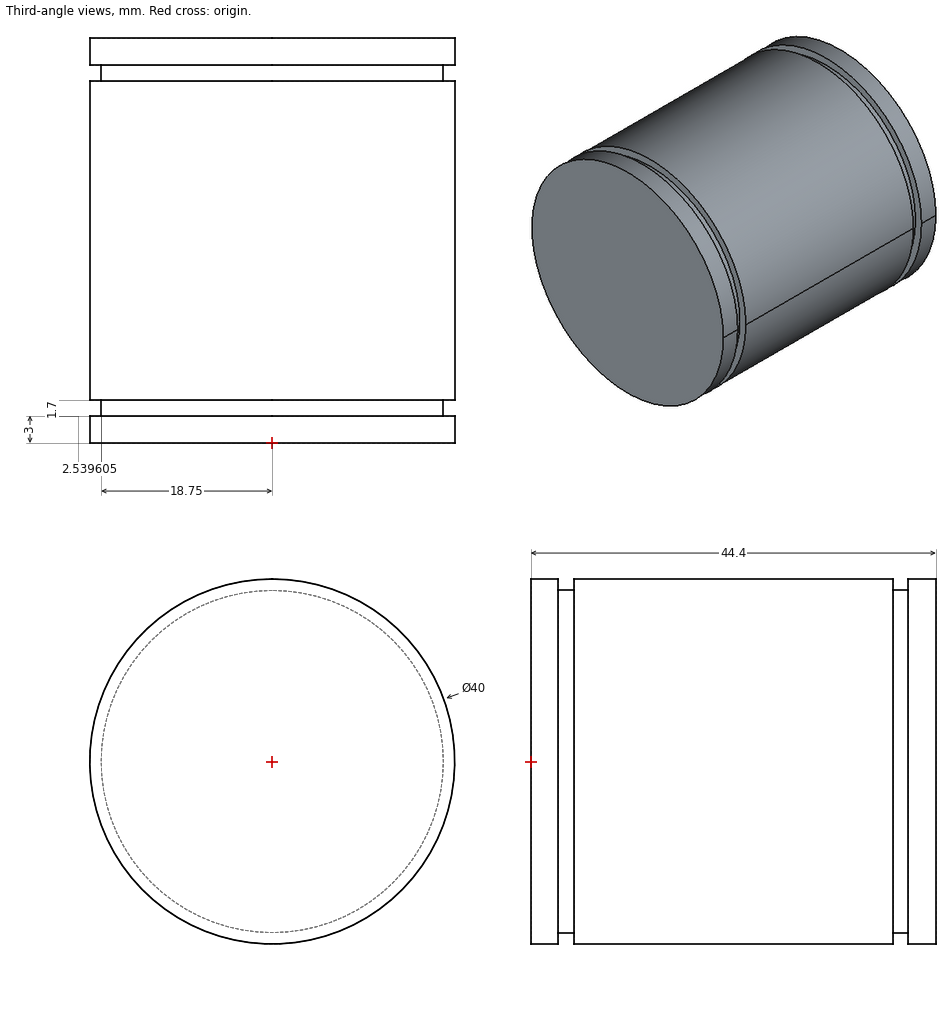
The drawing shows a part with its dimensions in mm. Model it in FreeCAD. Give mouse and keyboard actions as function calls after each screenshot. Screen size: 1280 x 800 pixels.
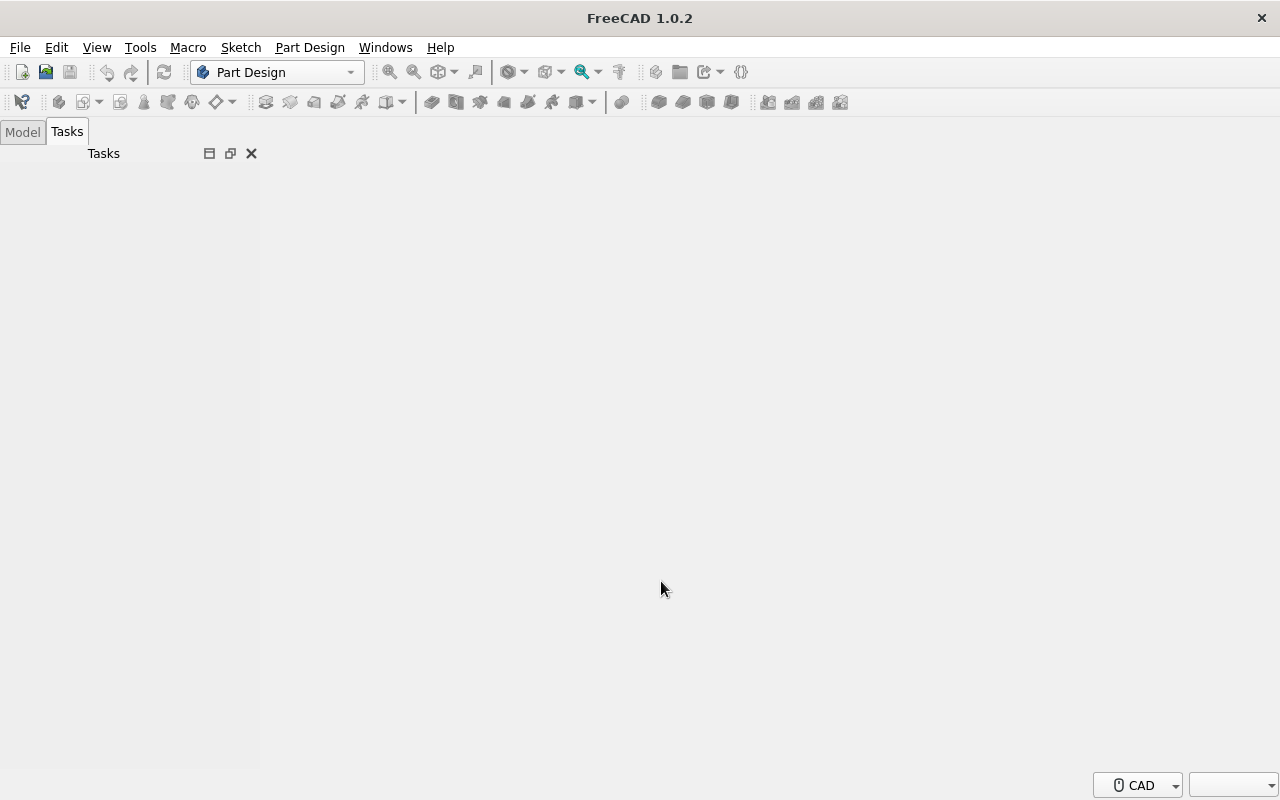
key(ctrl+n)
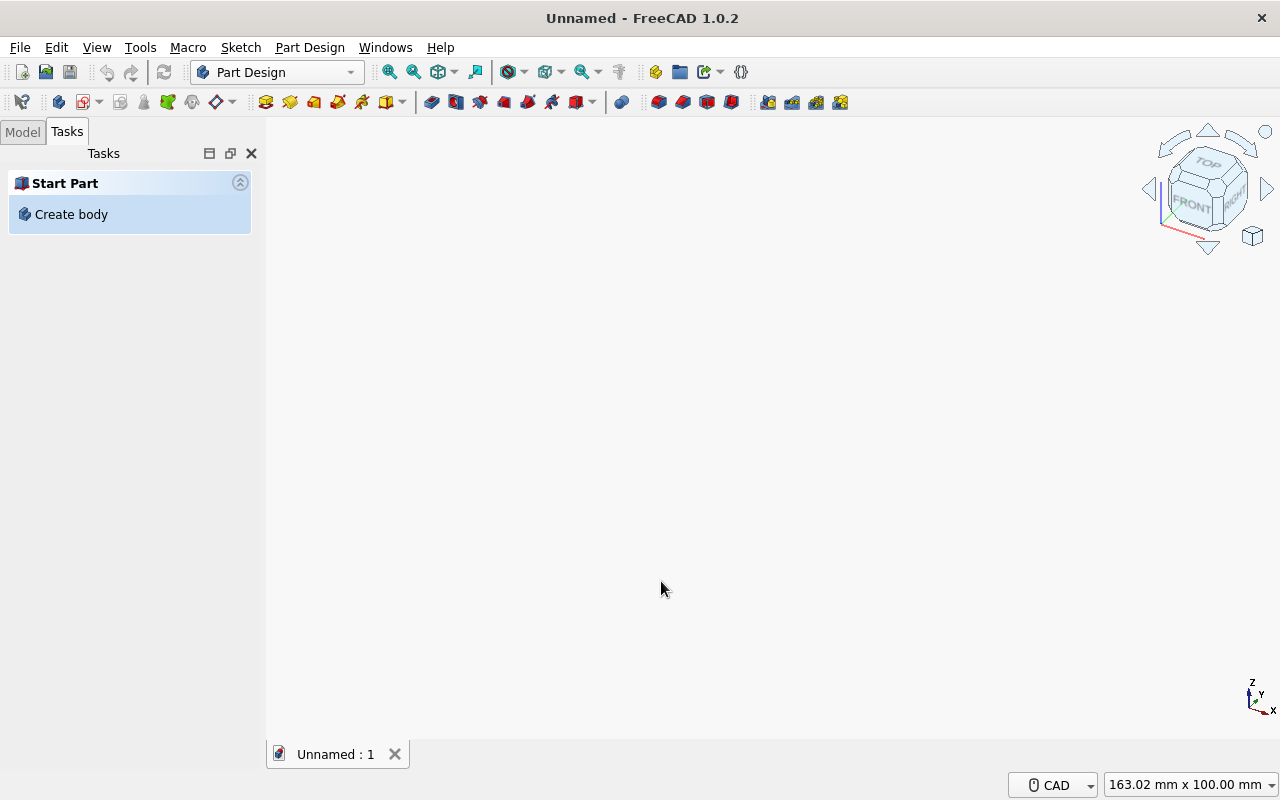
click(84, 102)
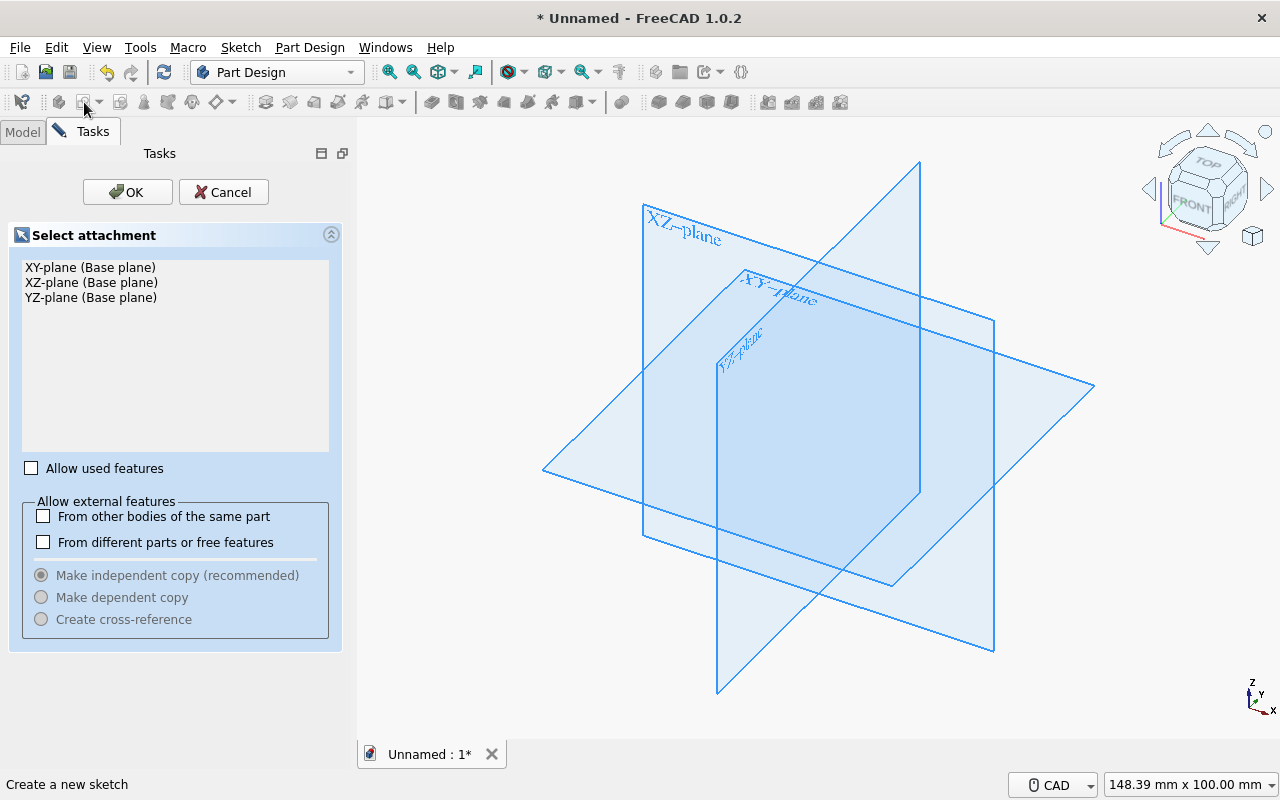
click(82, 282)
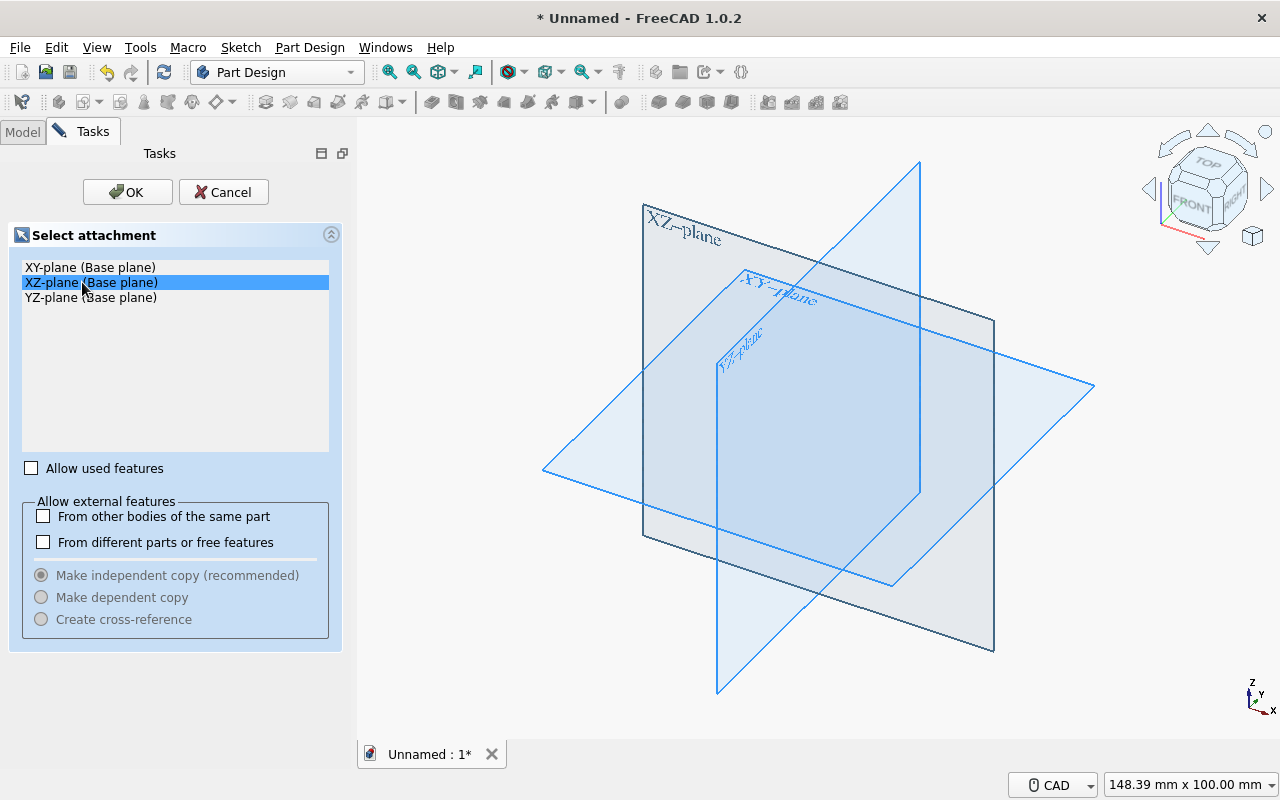
click(128, 192)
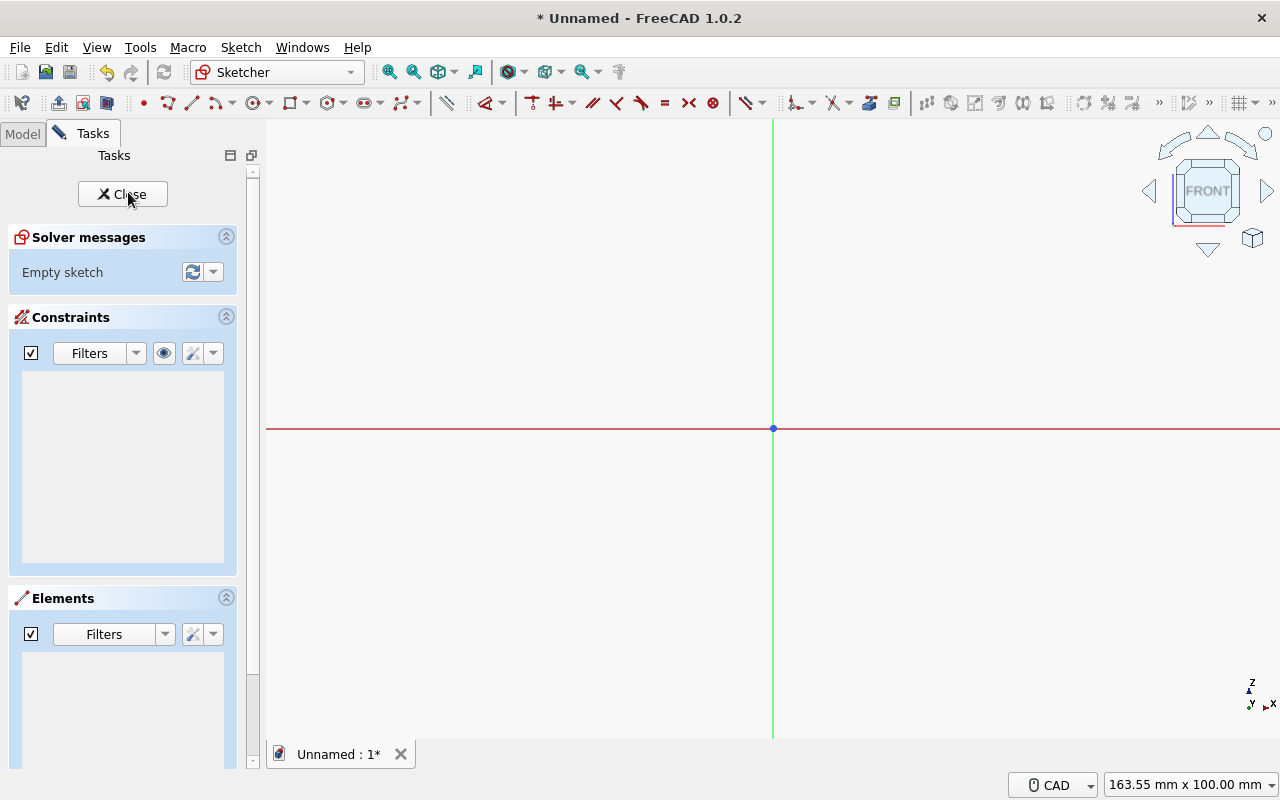
scroll(912, 429, up, 2)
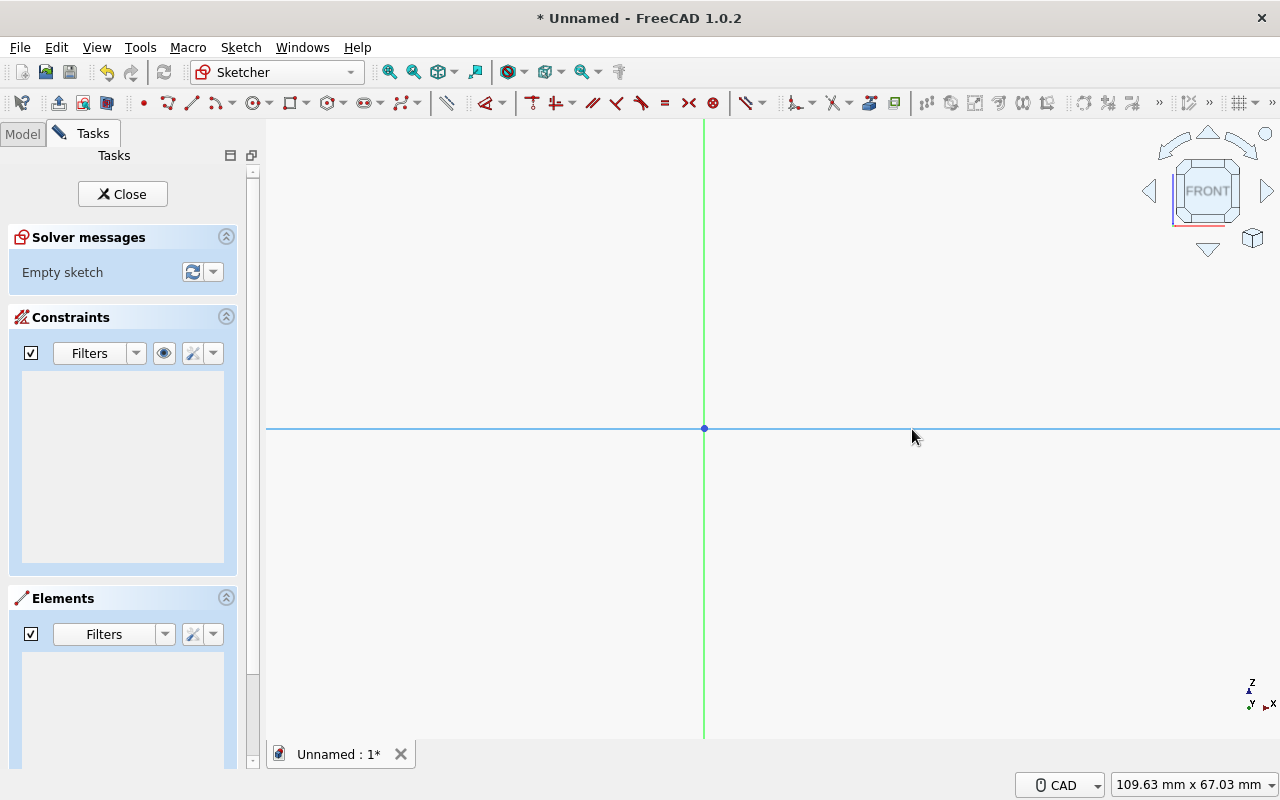
click(254, 104)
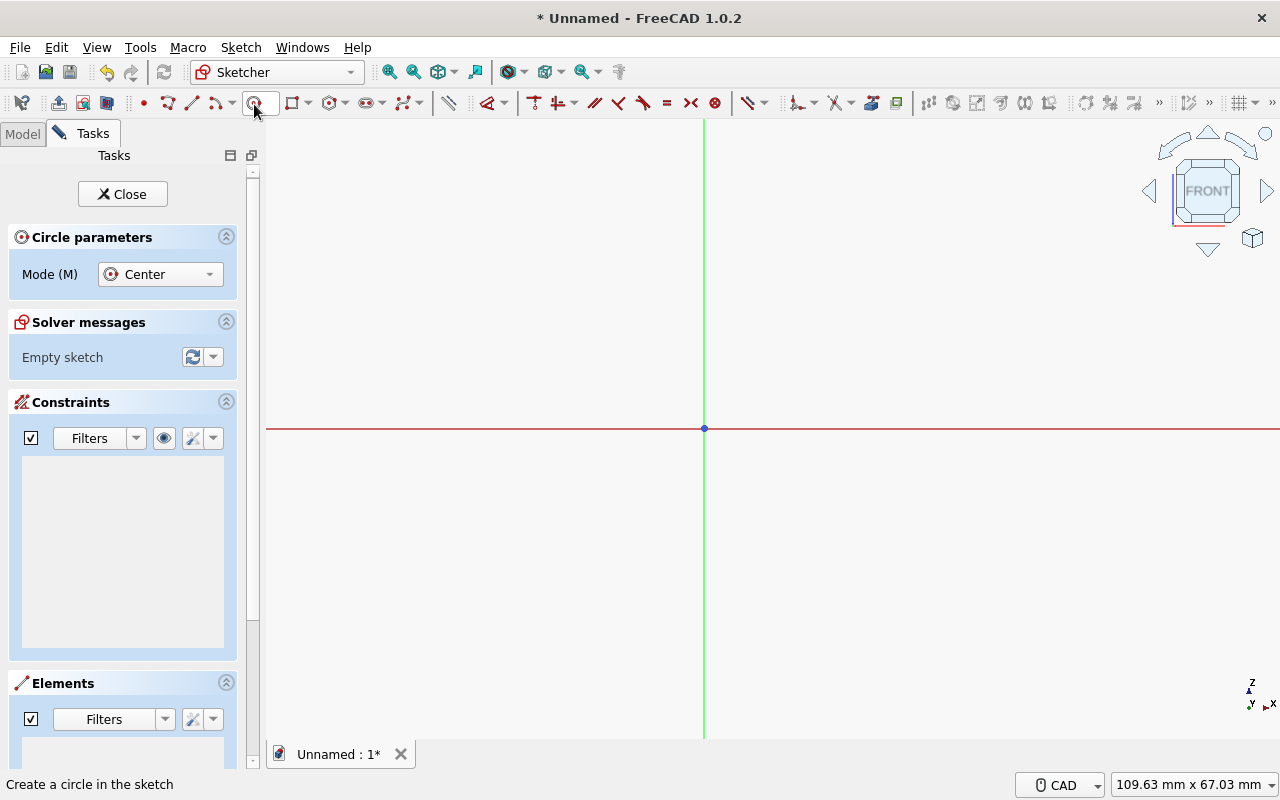
click(704, 429)
move(835, 298)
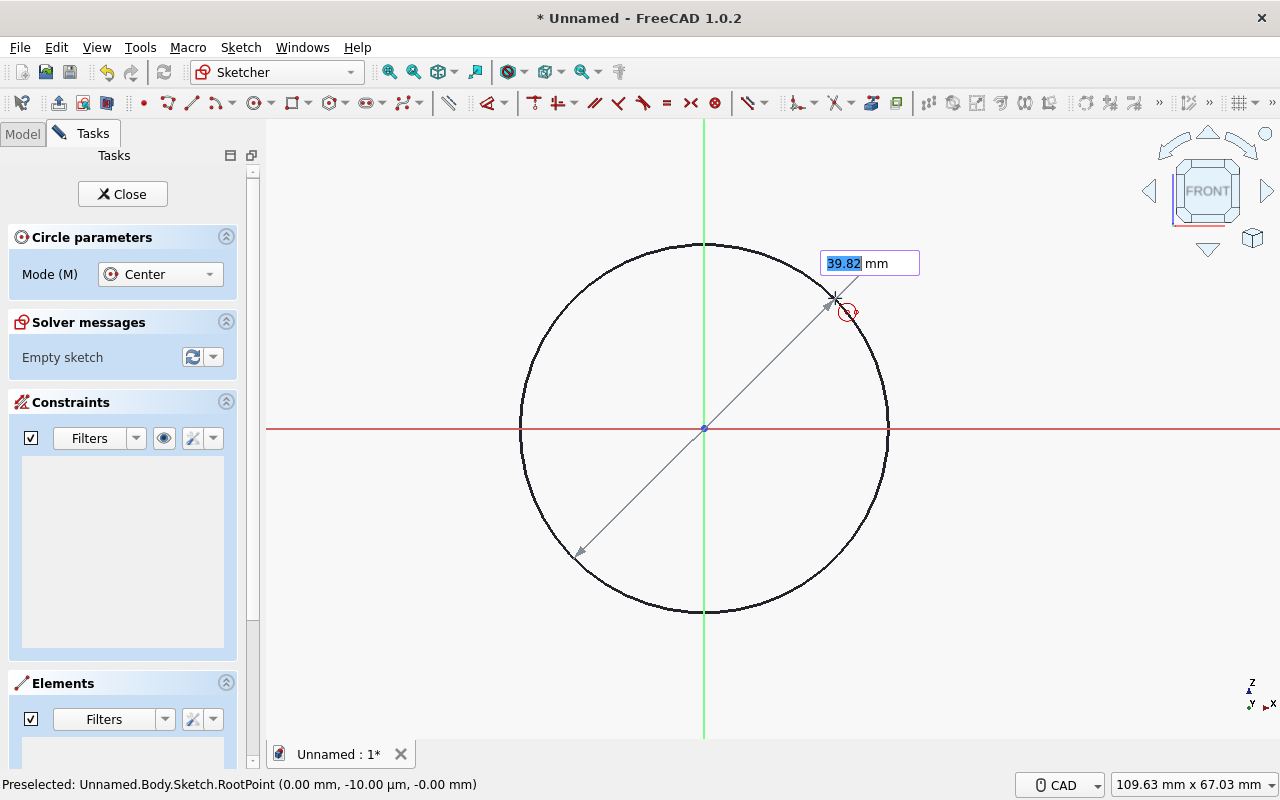
text(40)
key(Return)
key(Escape)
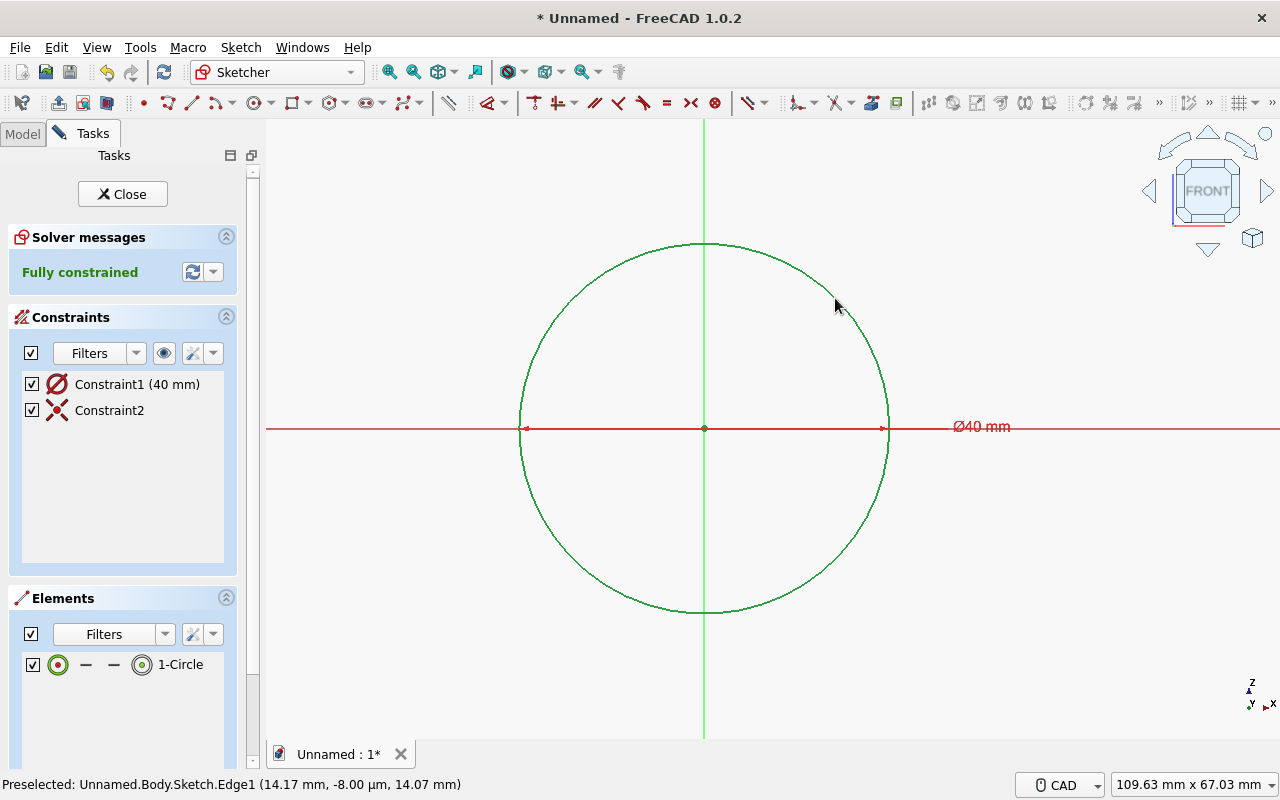
click(123, 194)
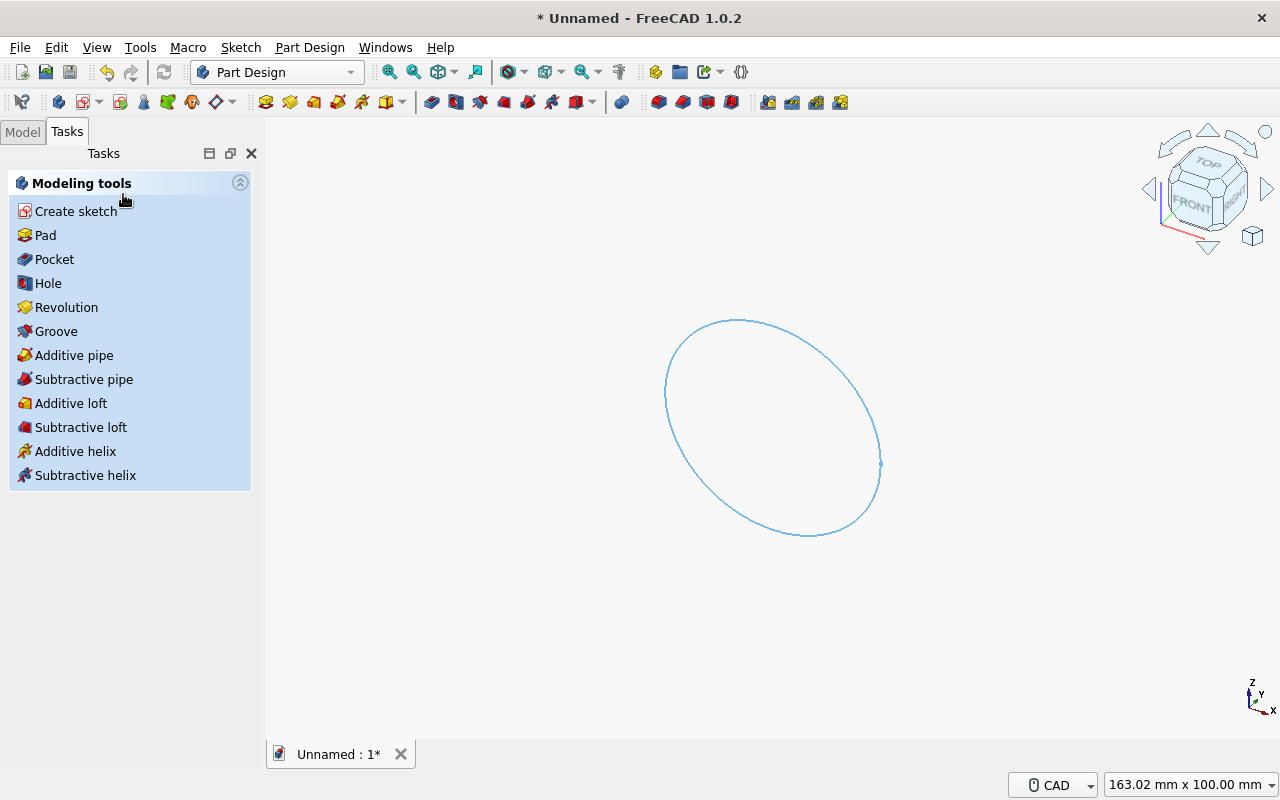
click(266, 102)